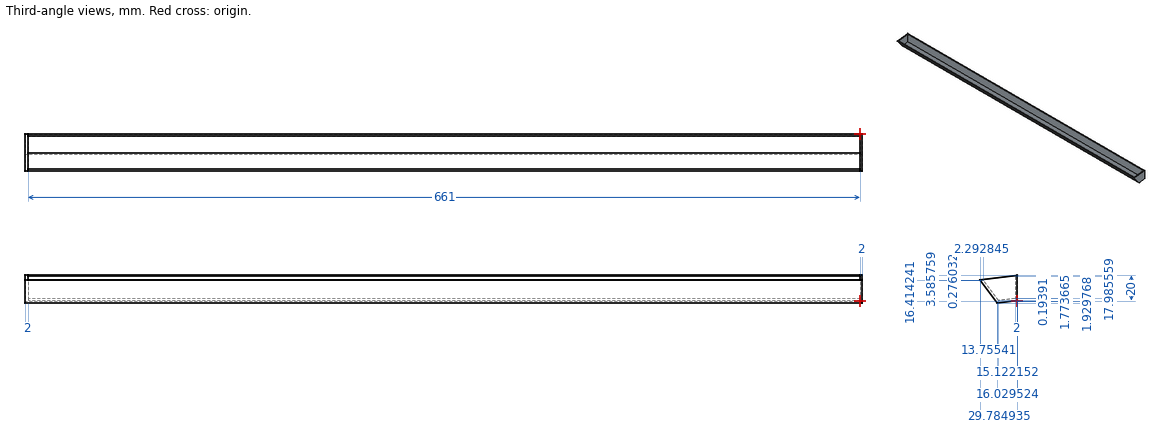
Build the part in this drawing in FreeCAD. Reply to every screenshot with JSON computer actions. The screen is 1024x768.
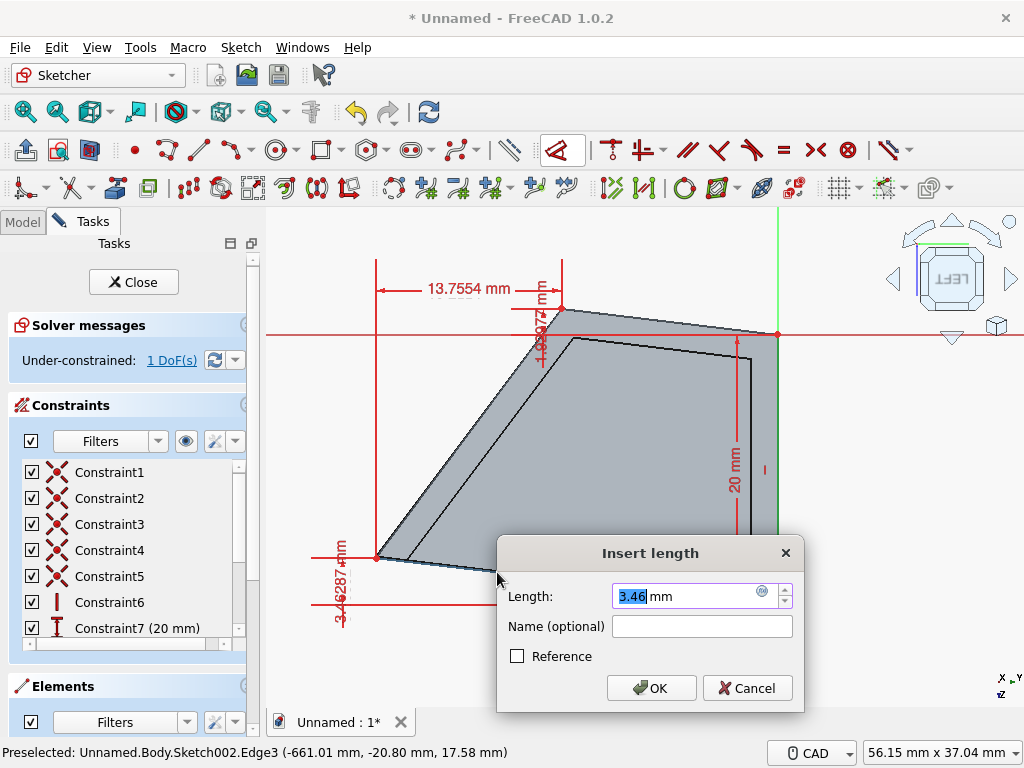
{"action": "type", "text": "3.585759"}
{"action": "key", "text": "Return"}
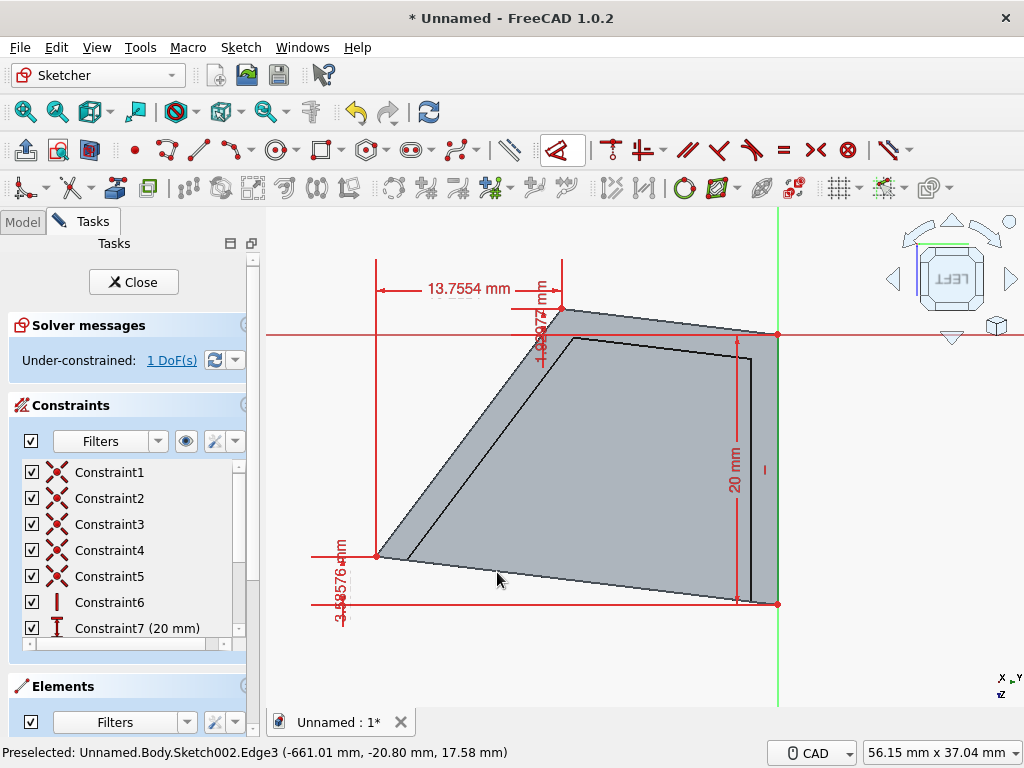
{"action": "left_click", "coordinate": [562, 309]}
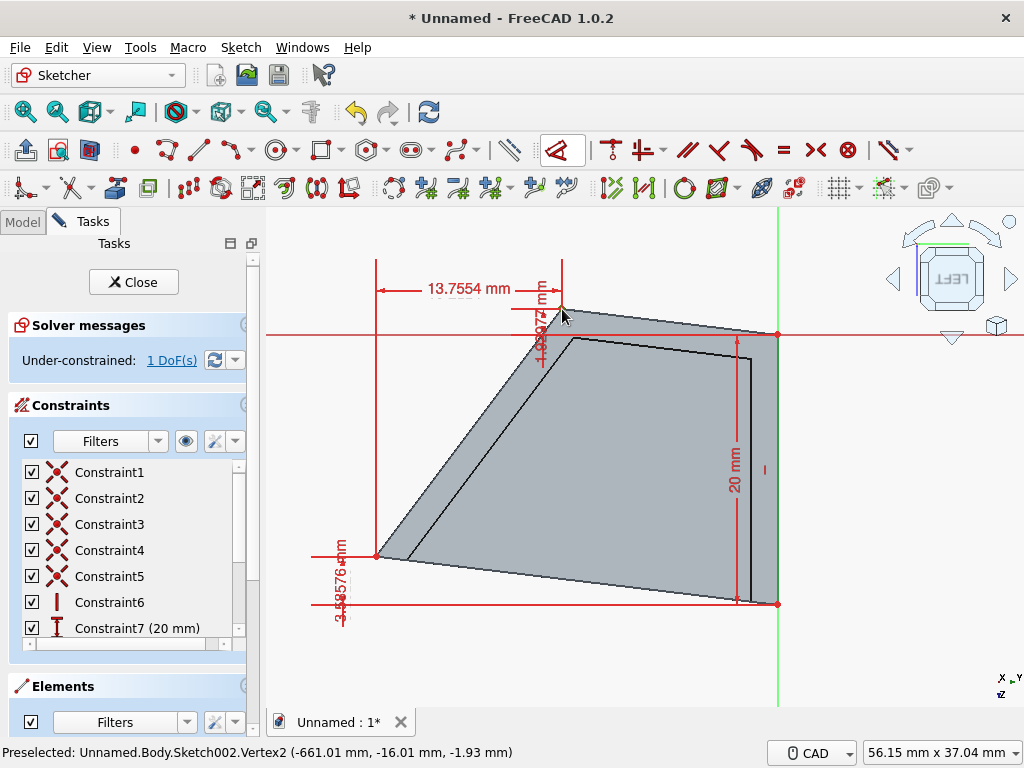
{"action": "left_click", "coordinate": [580, 150]}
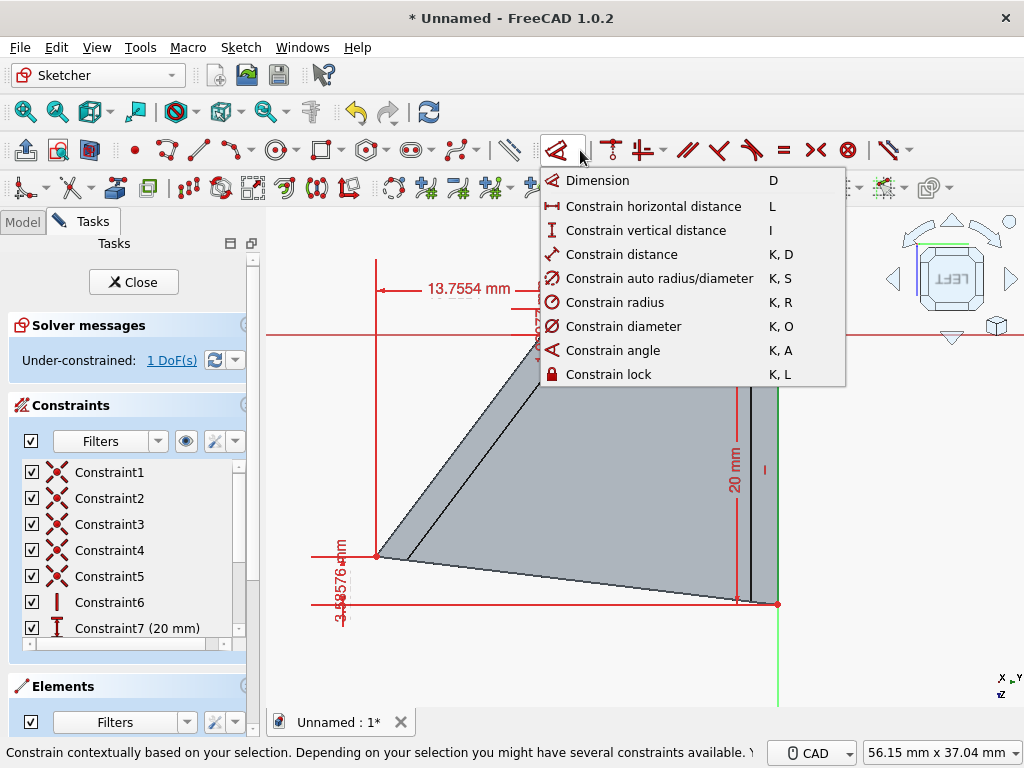
{"action": "left_click", "coordinate": [693, 206]}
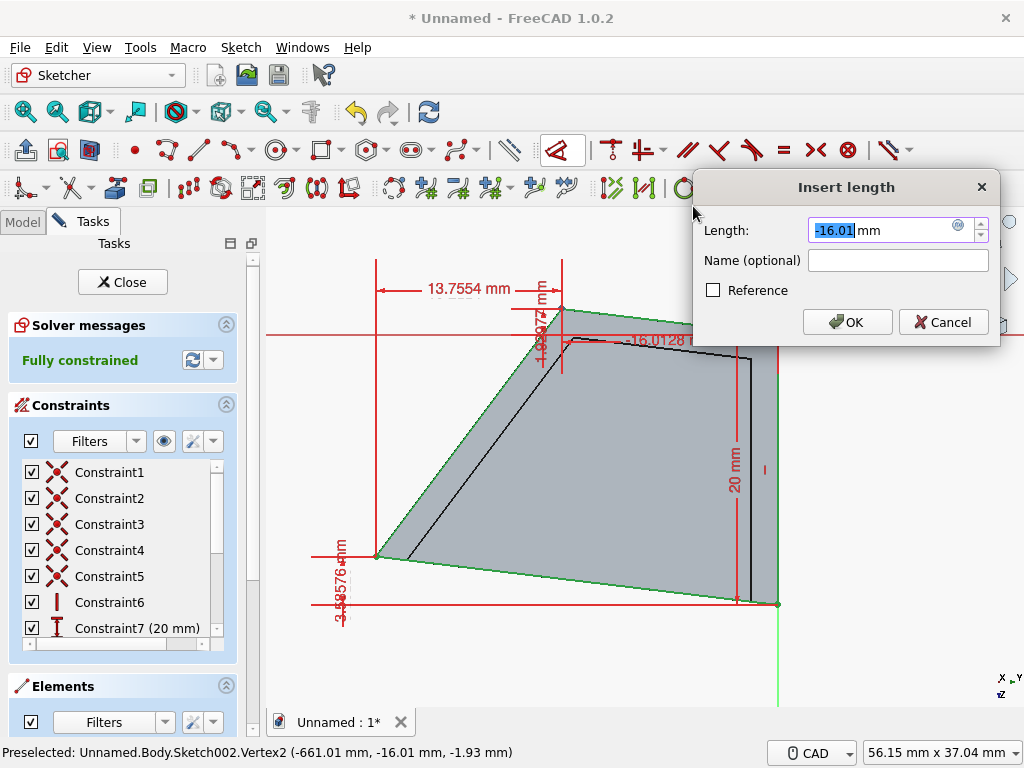
{"action": "type", "text": "-16.029524"}
{"action": "key", "text": "Return"}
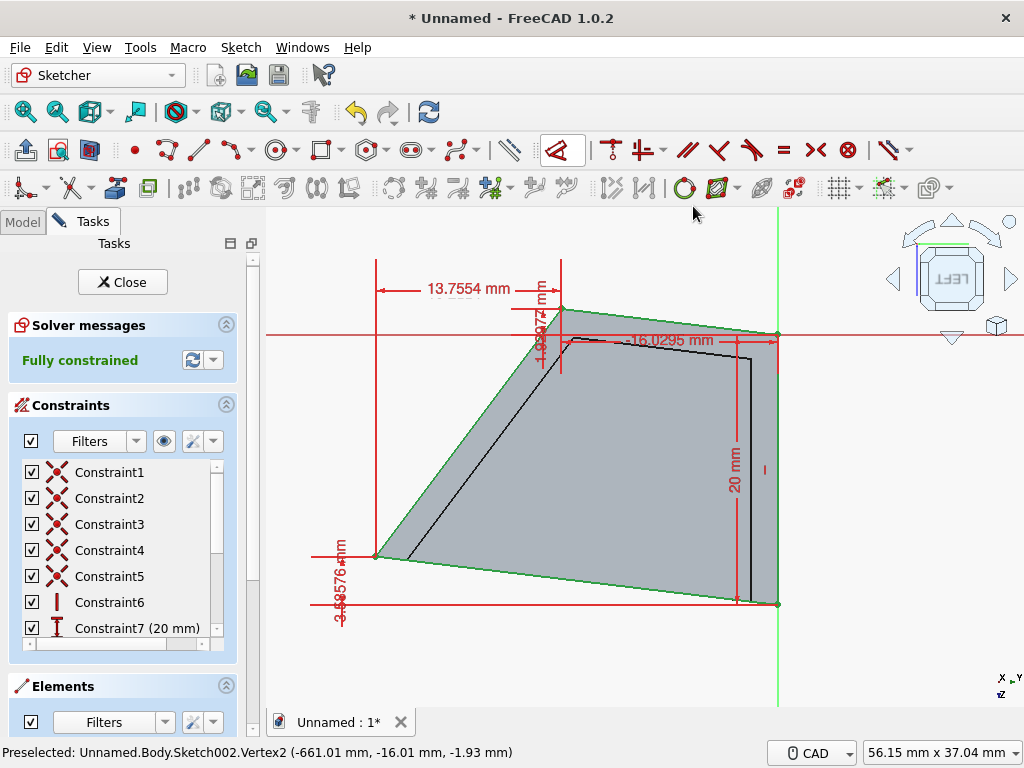
{"action": "left_click", "coordinate": [123, 282]}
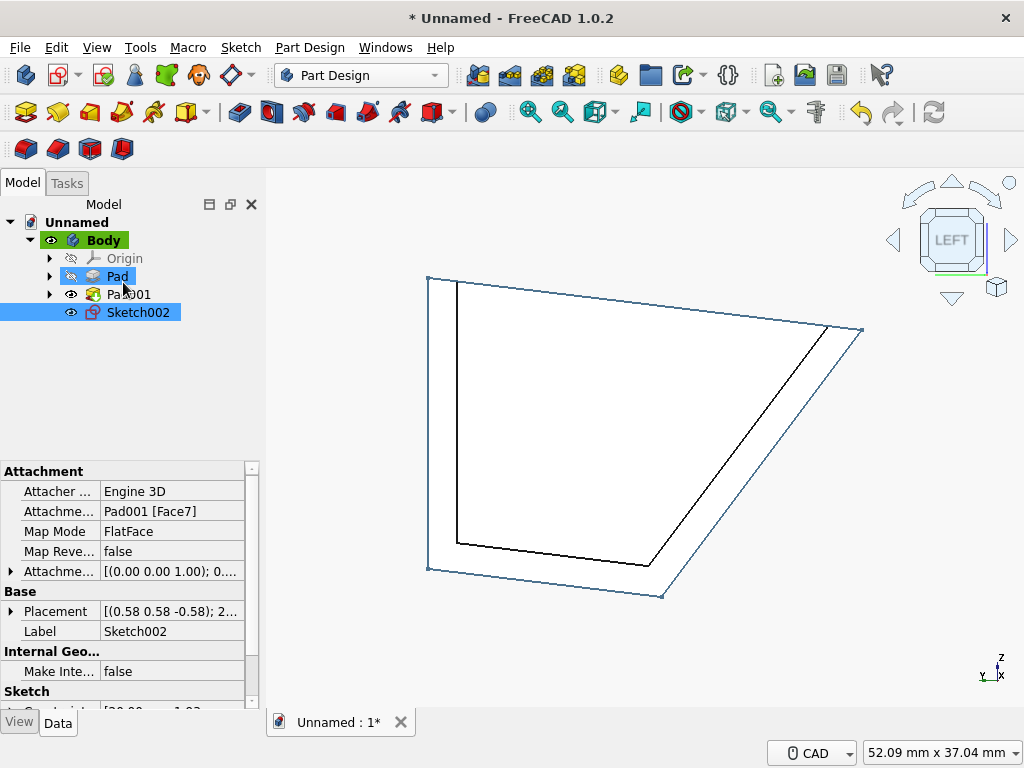
{"action": "left_click", "coordinate": [26, 112]}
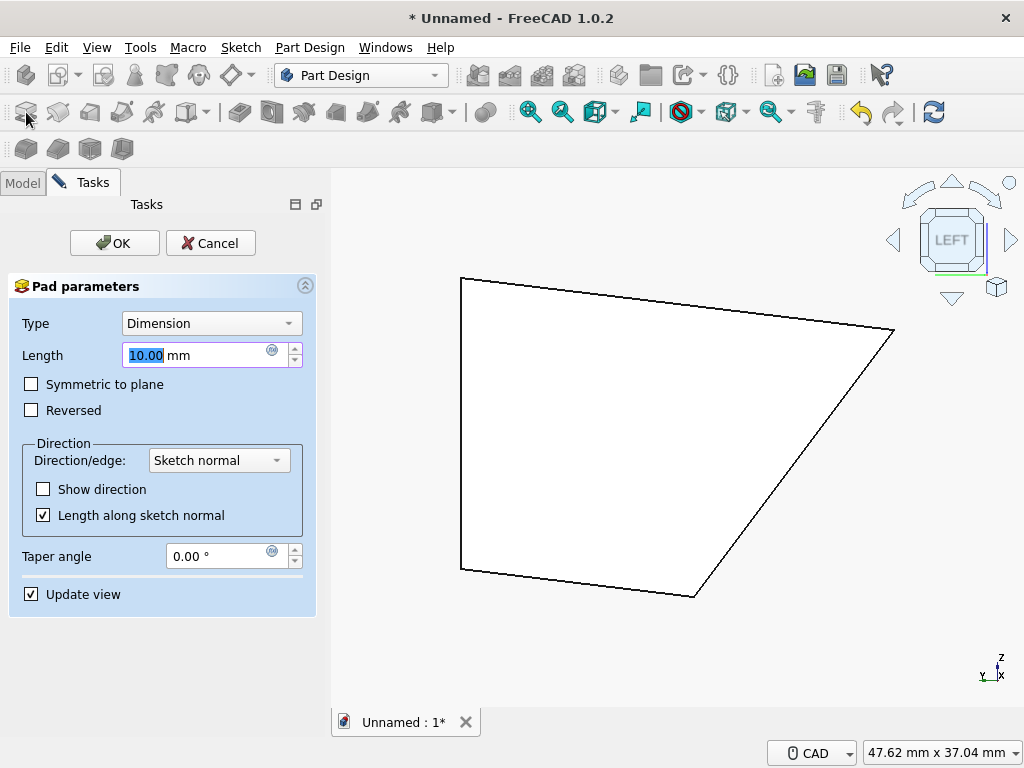
{"action": "type", "text": "2"}
{"action": "key", "text": "Tab"}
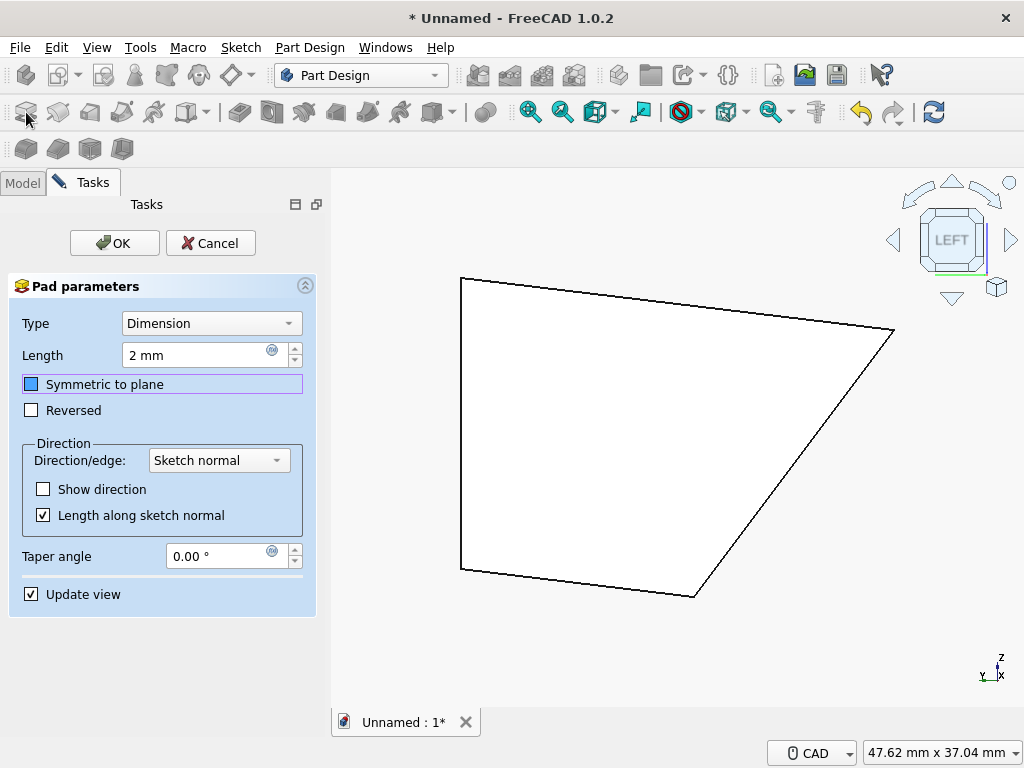
{"action": "left_click", "coordinate": [115, 243]}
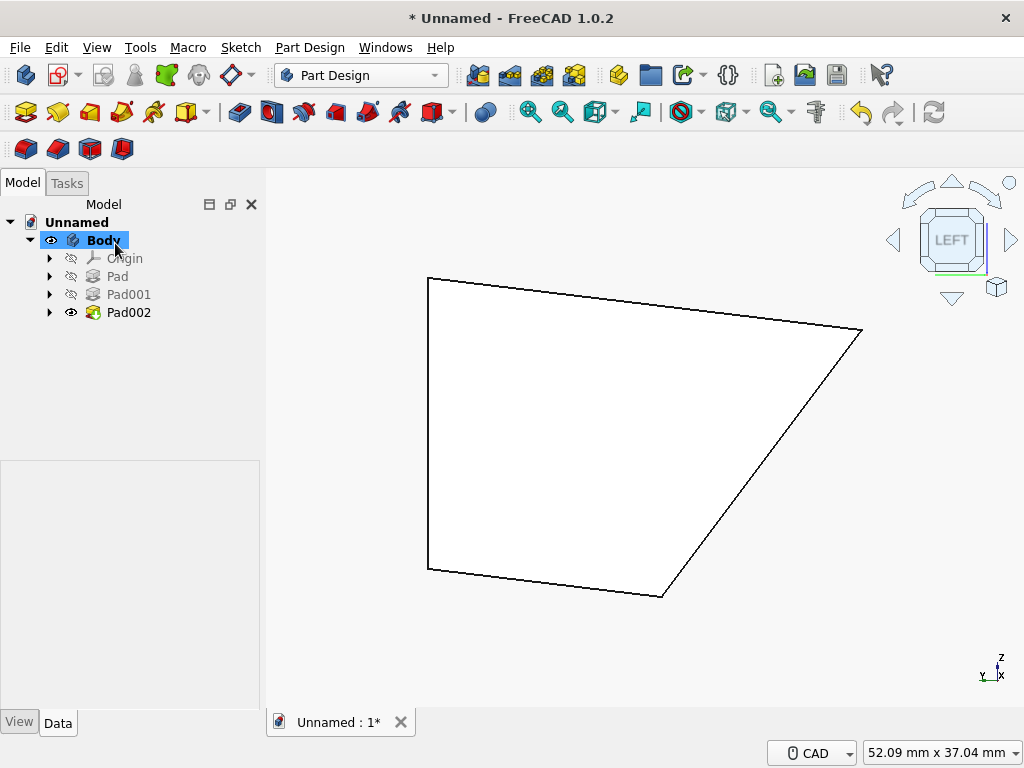
{"action": "key", "text": "0"}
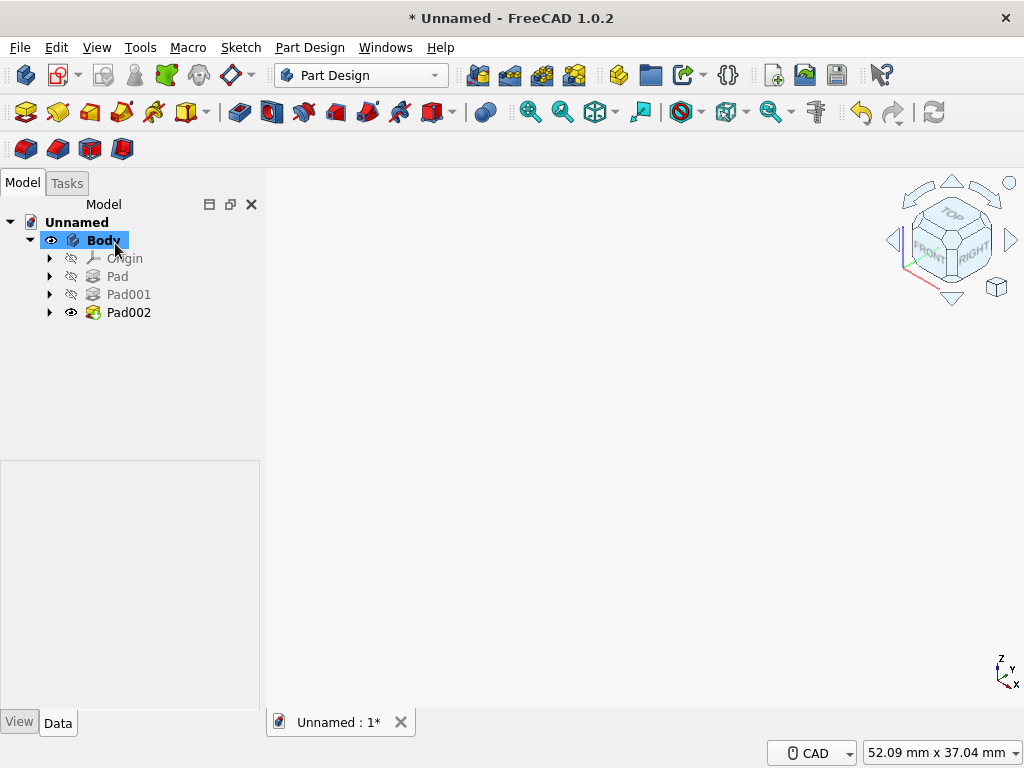
{"action": "left_click", "coordinate": [532, 112]}